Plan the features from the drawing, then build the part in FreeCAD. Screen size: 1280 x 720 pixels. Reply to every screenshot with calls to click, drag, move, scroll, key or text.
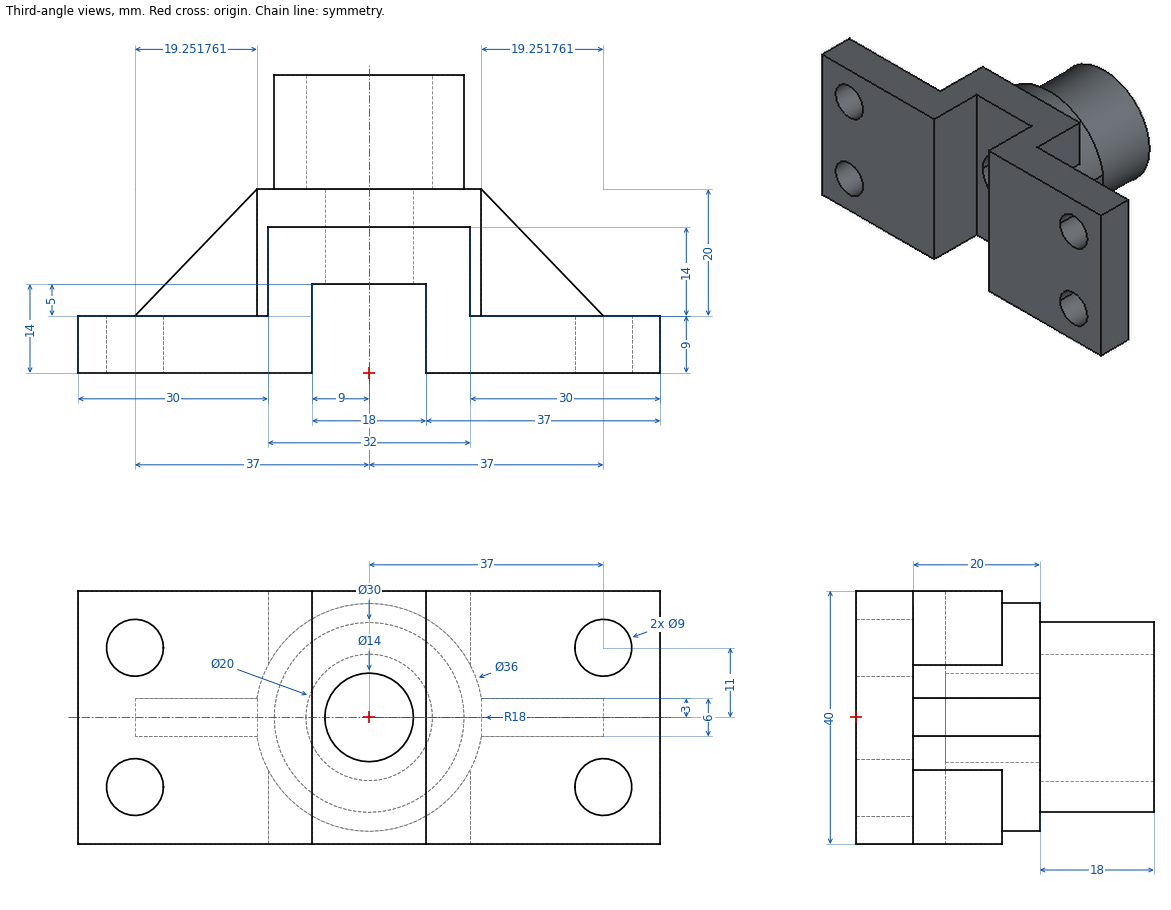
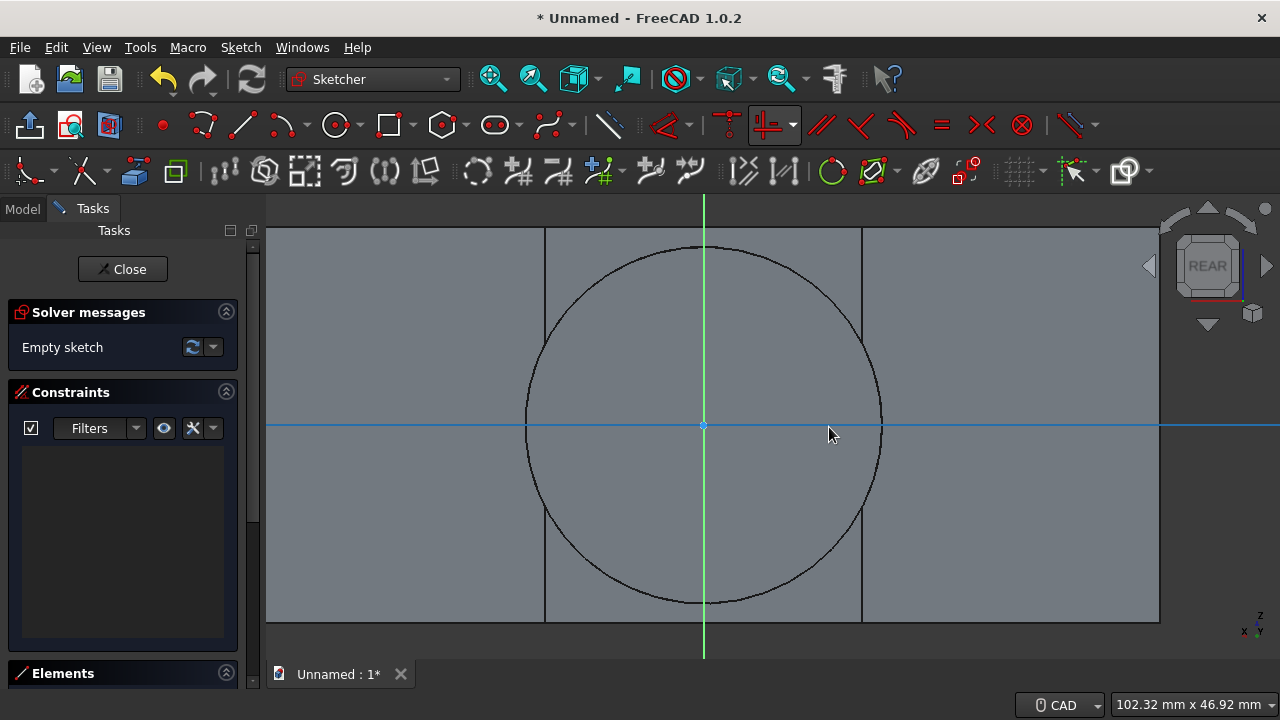
key(g)
key(c)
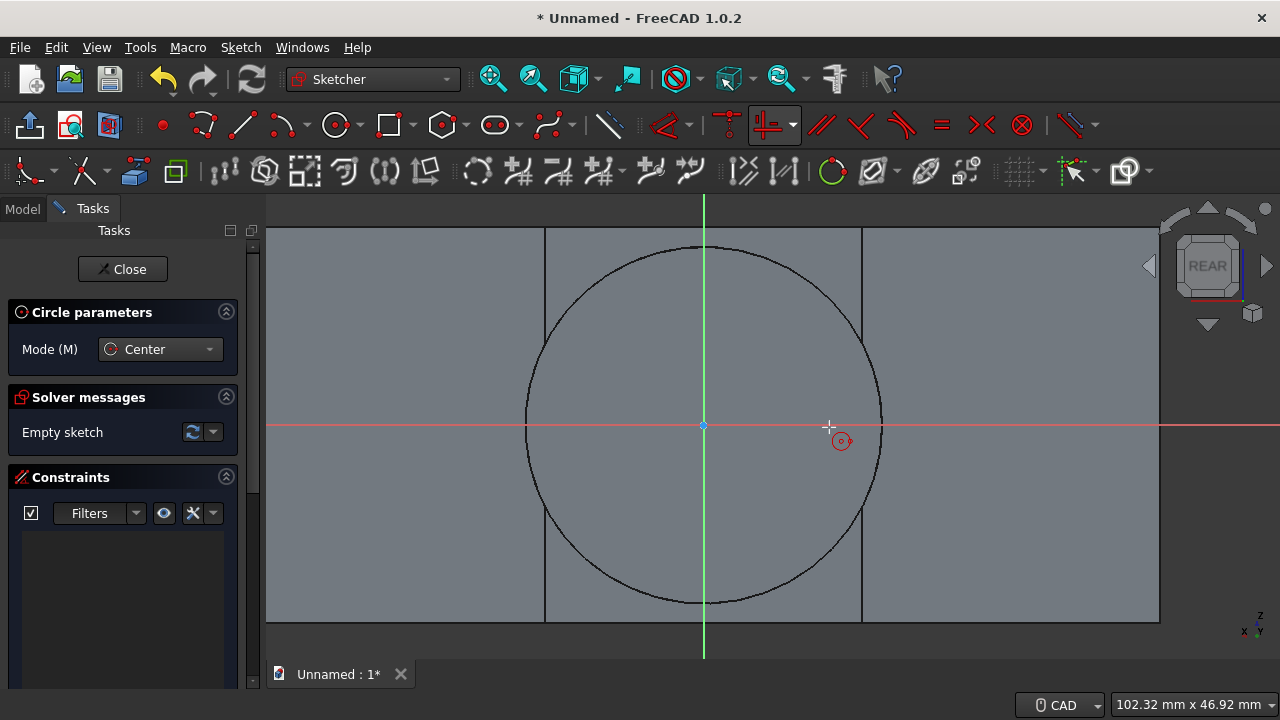
click(704, 425)
click(809, 320)
key(Escape)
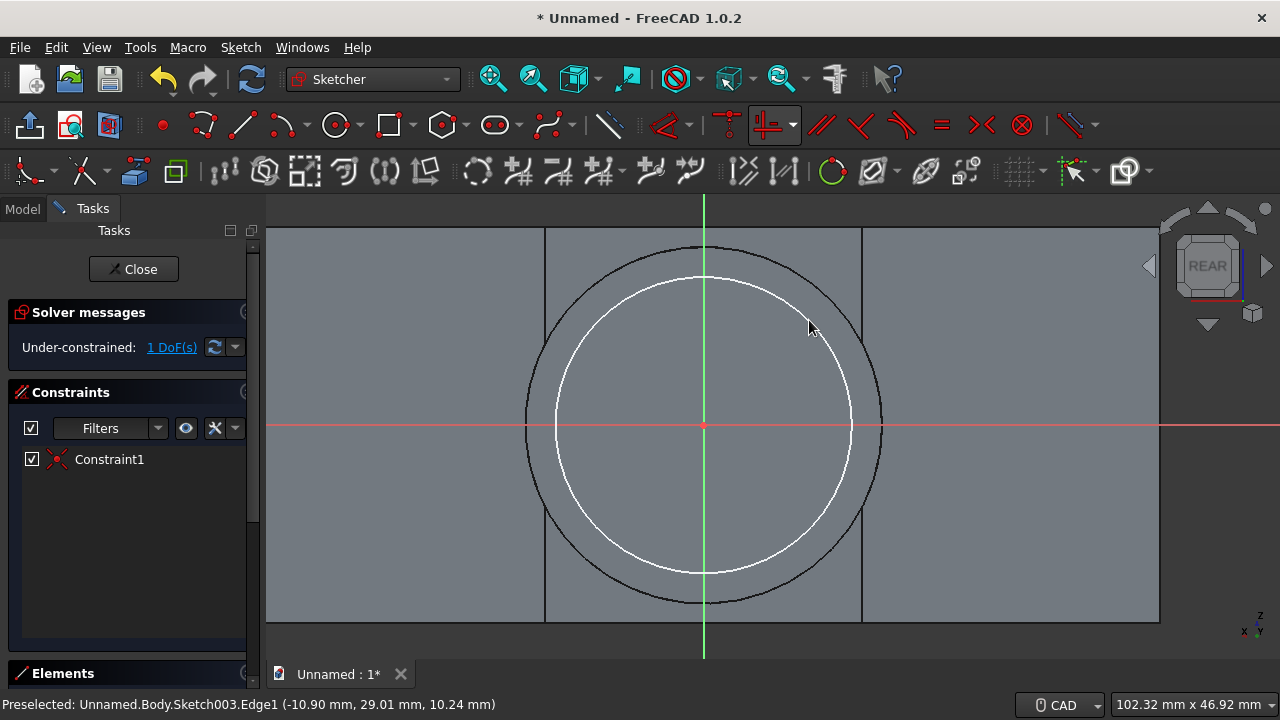
key(d)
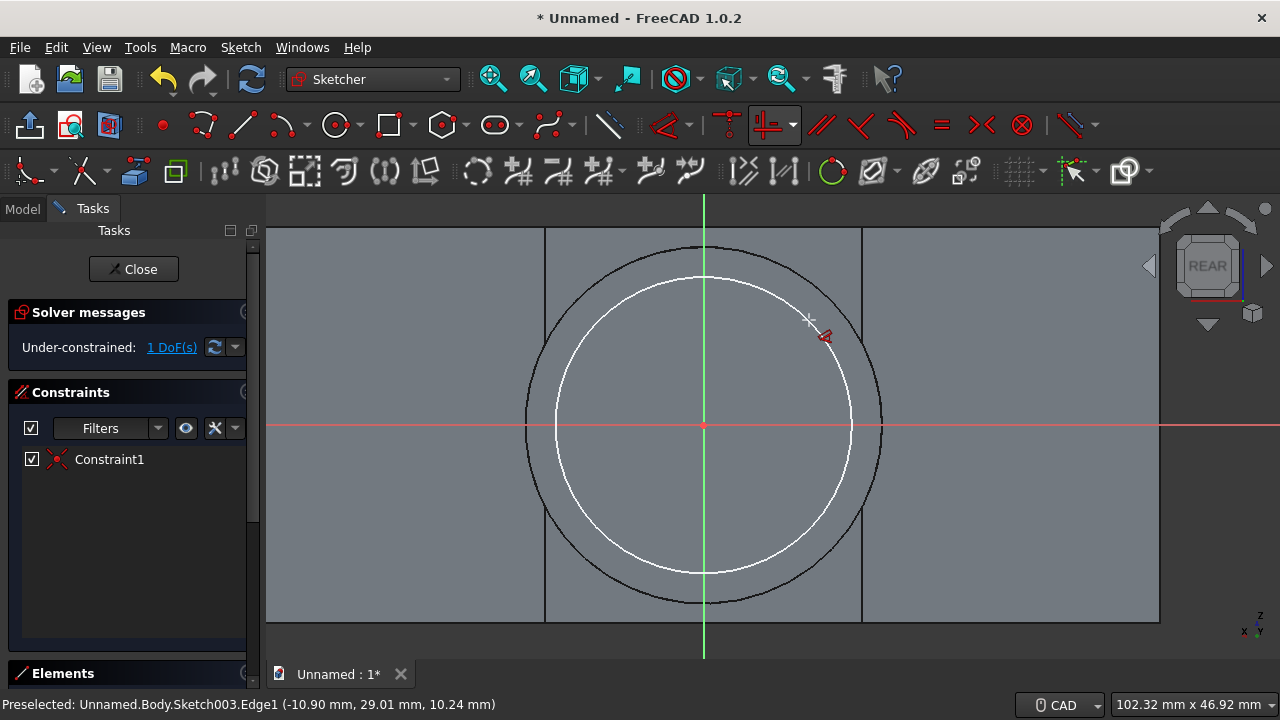
click(808, 320)
click(831, 297)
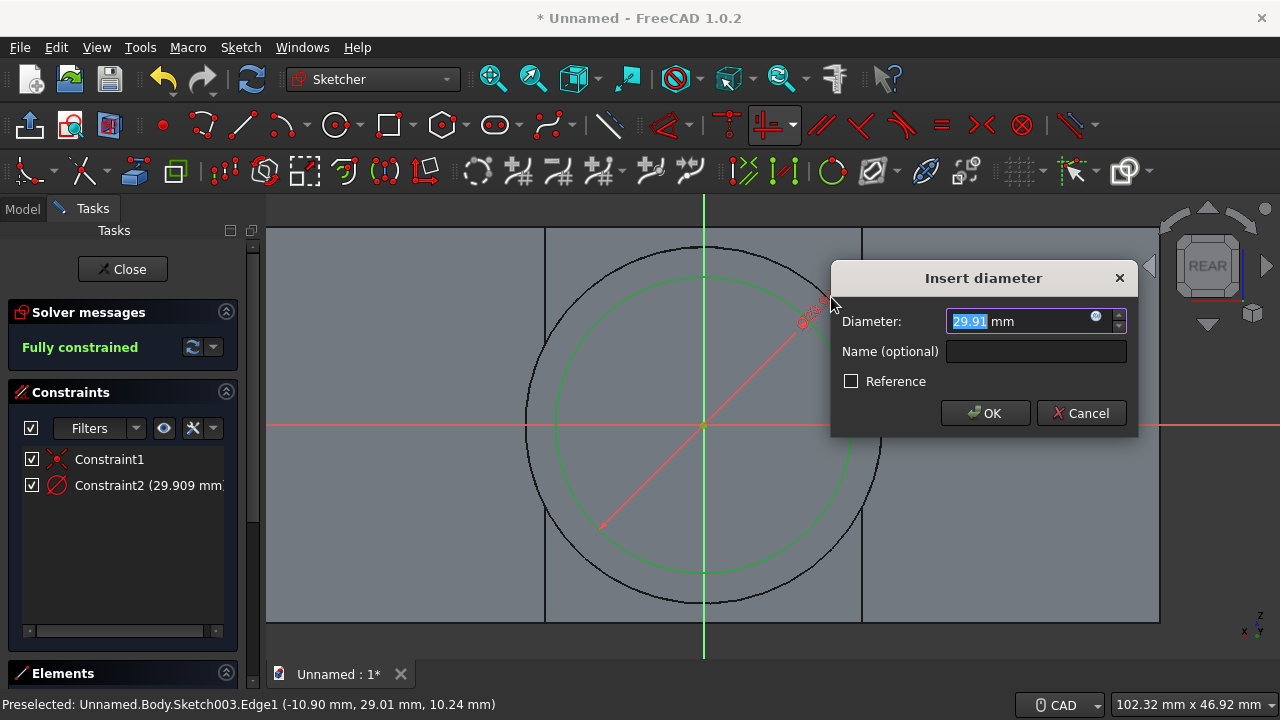
text(30)
key(Return)
key(Escape)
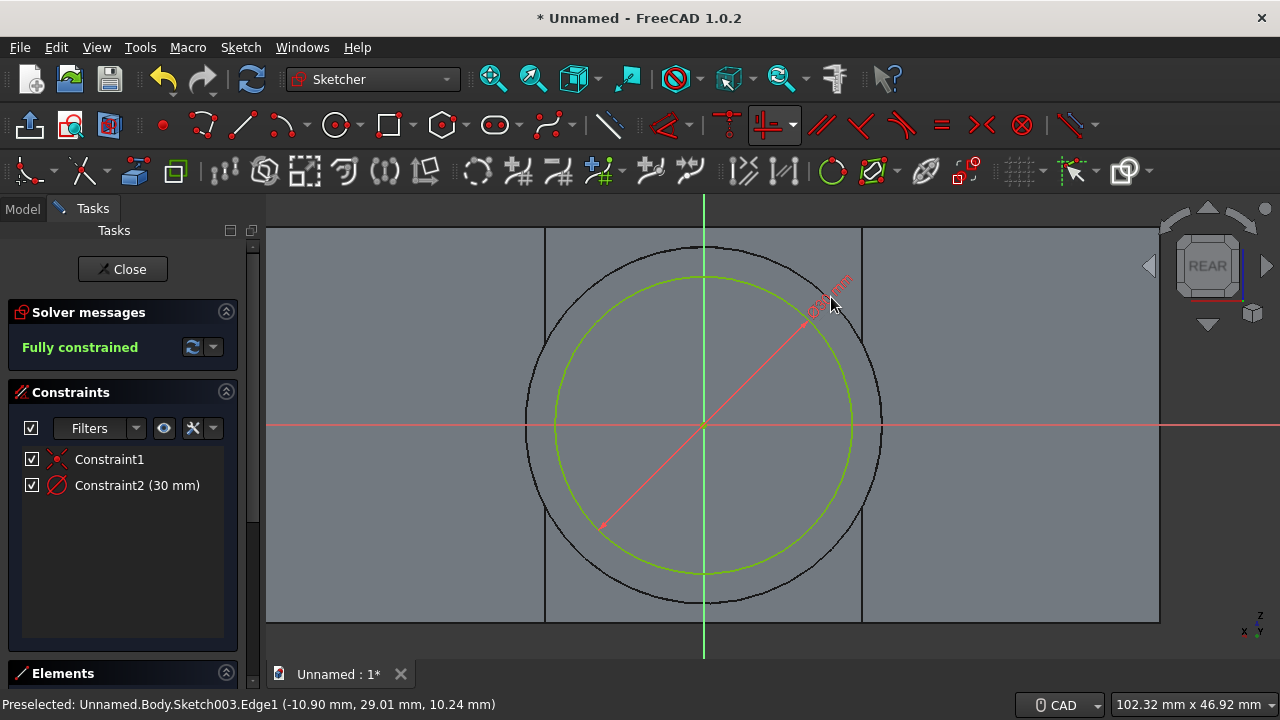
click(123, 269)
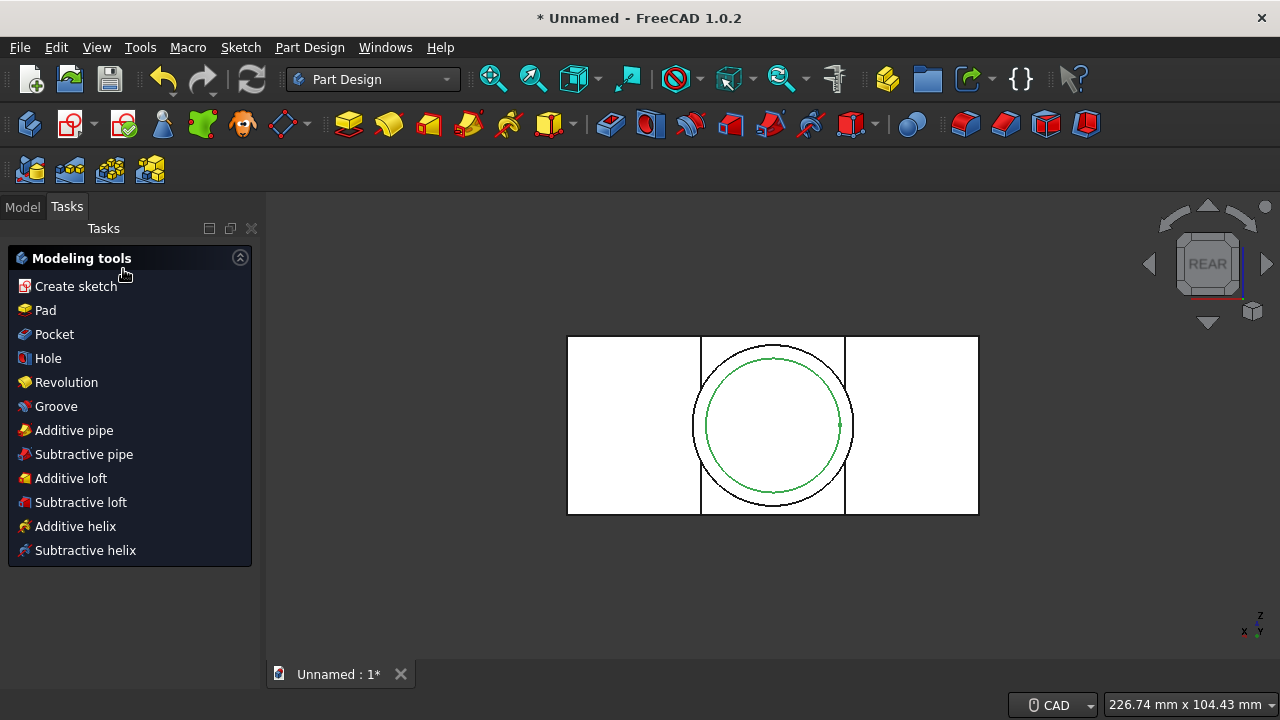
click(350, 124)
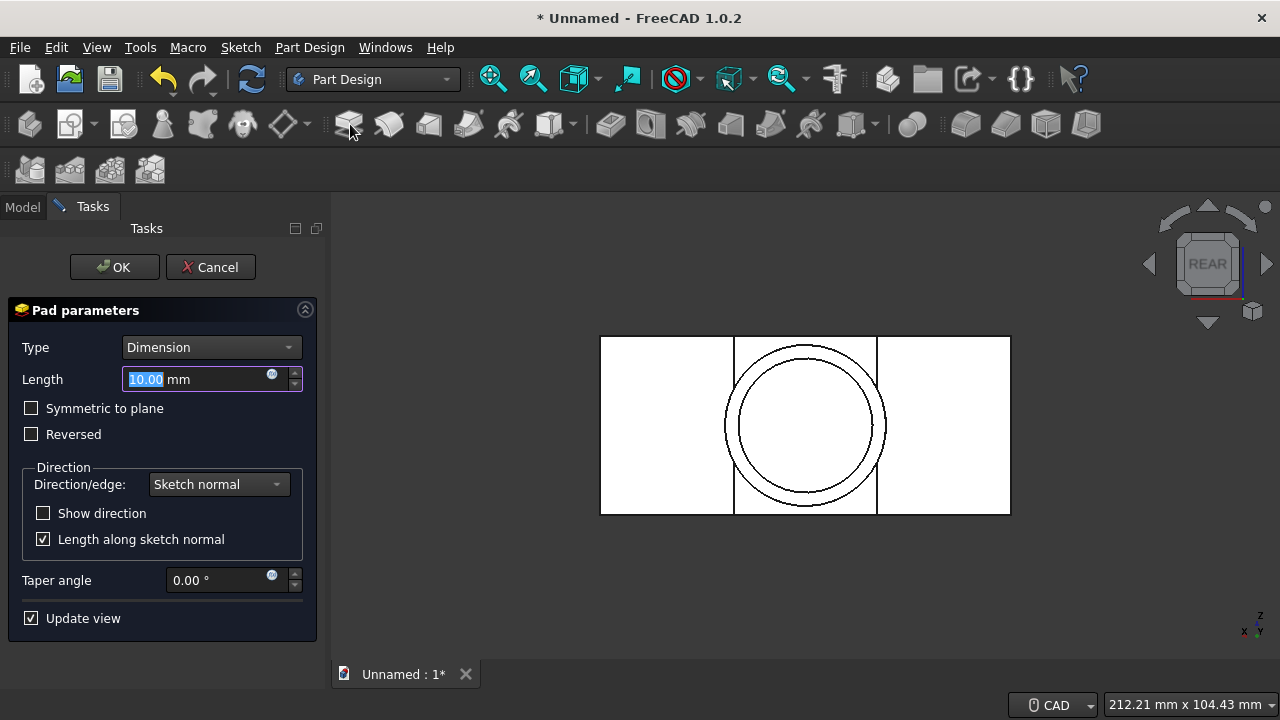
text(18)
key(Tab)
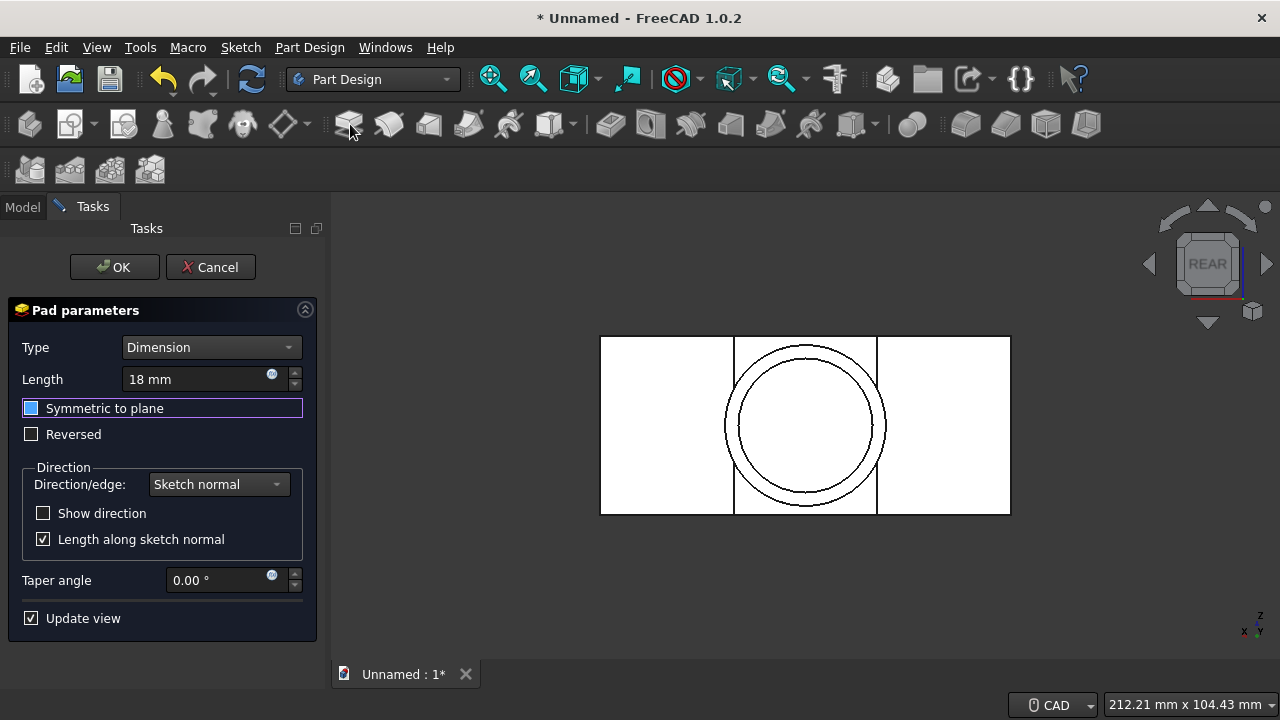
click(115, 267)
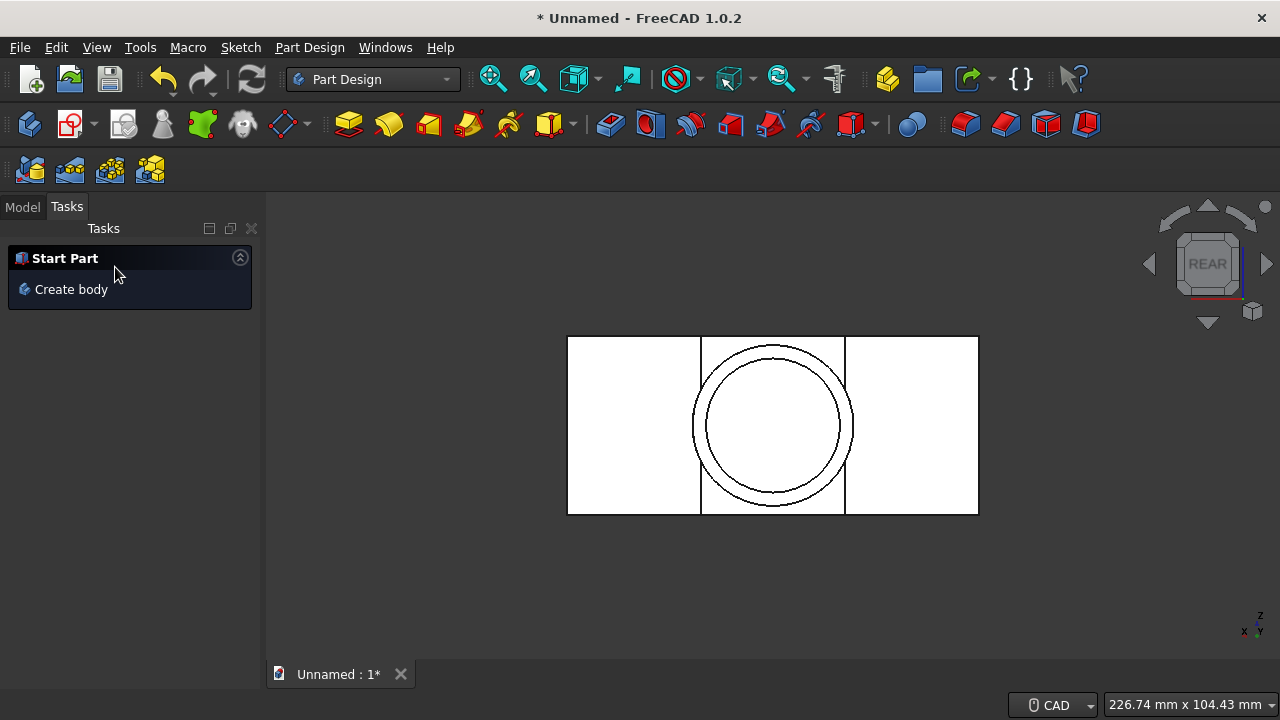
key(v)
key(f)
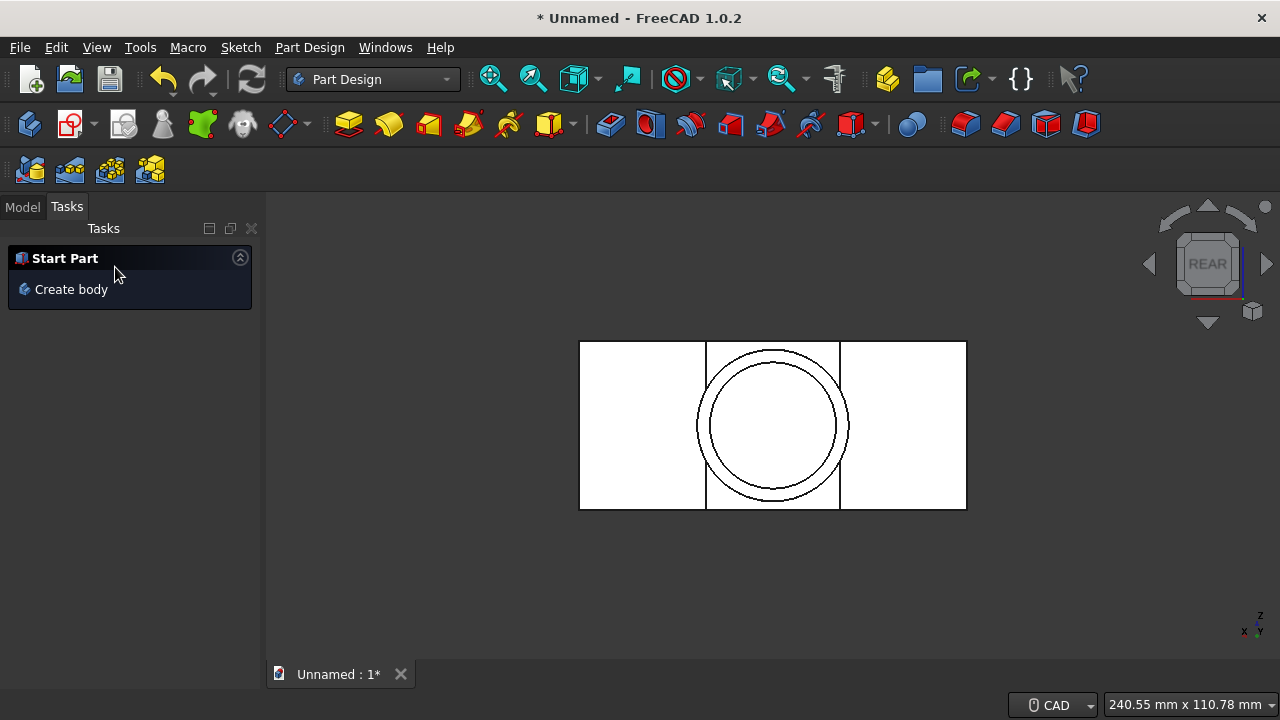
click(773, 424)